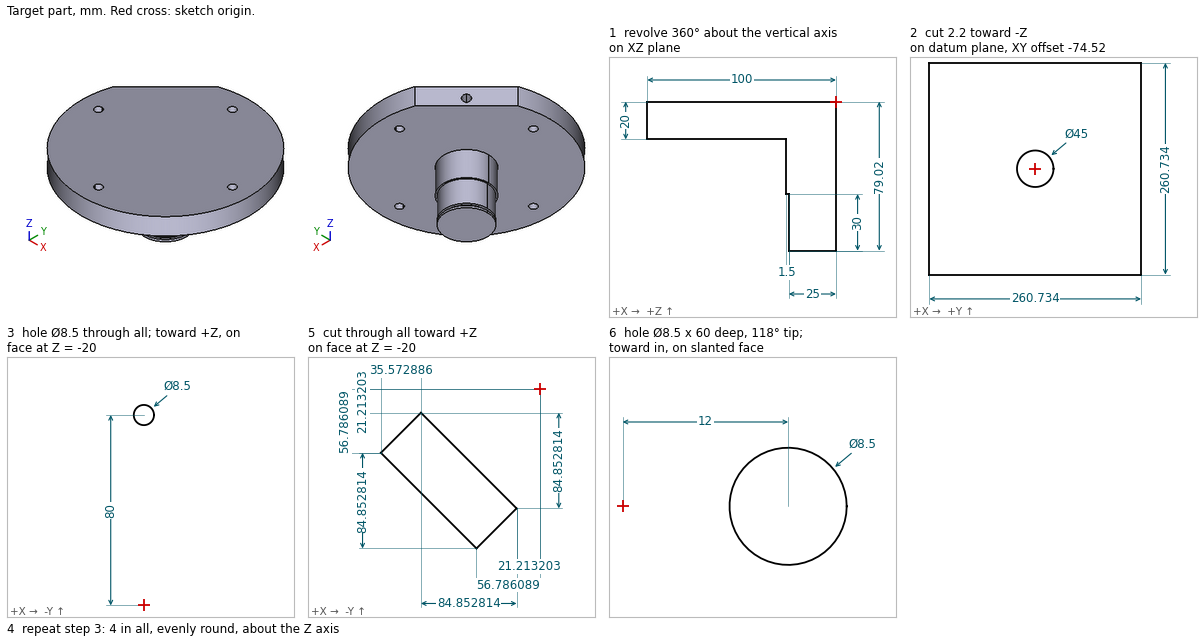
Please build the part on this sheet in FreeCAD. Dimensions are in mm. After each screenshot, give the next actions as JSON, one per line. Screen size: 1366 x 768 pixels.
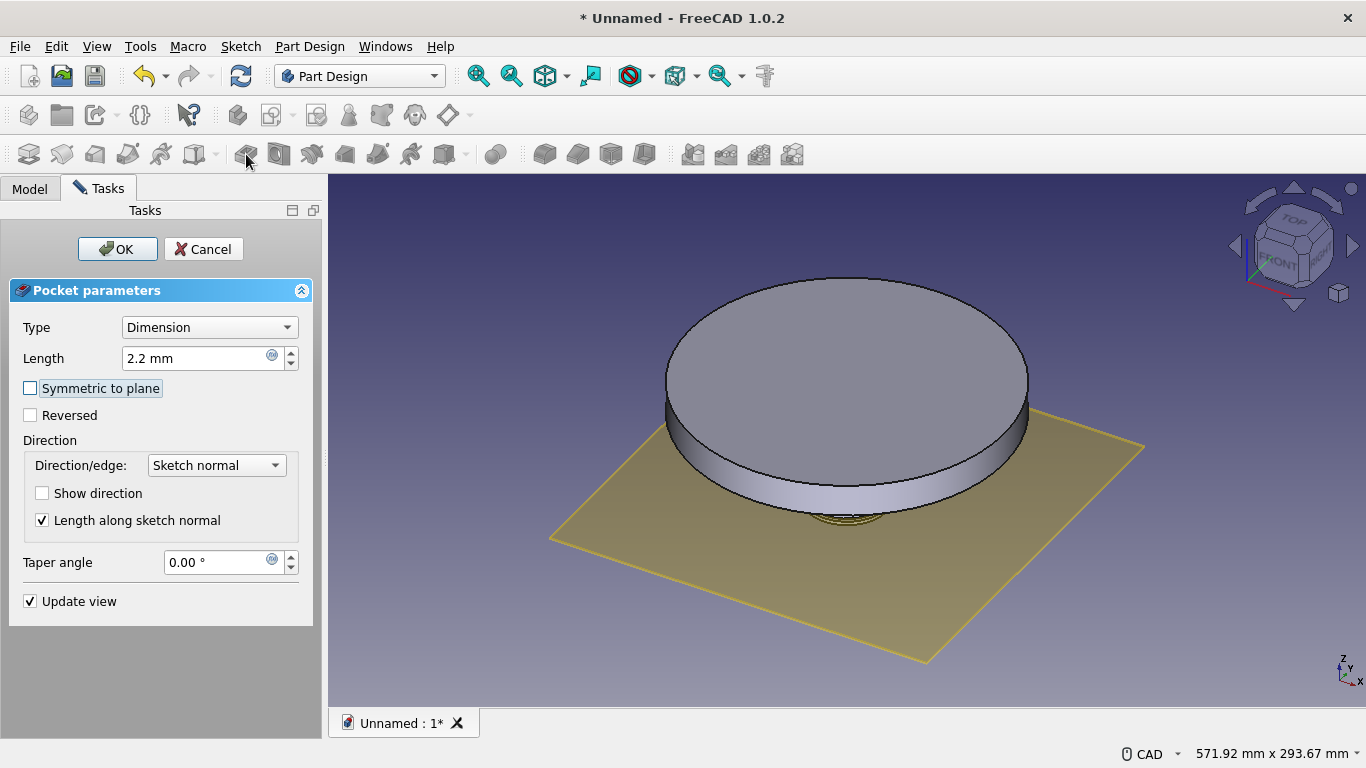
{"action": "left_click", "coordinate": [118, 249]}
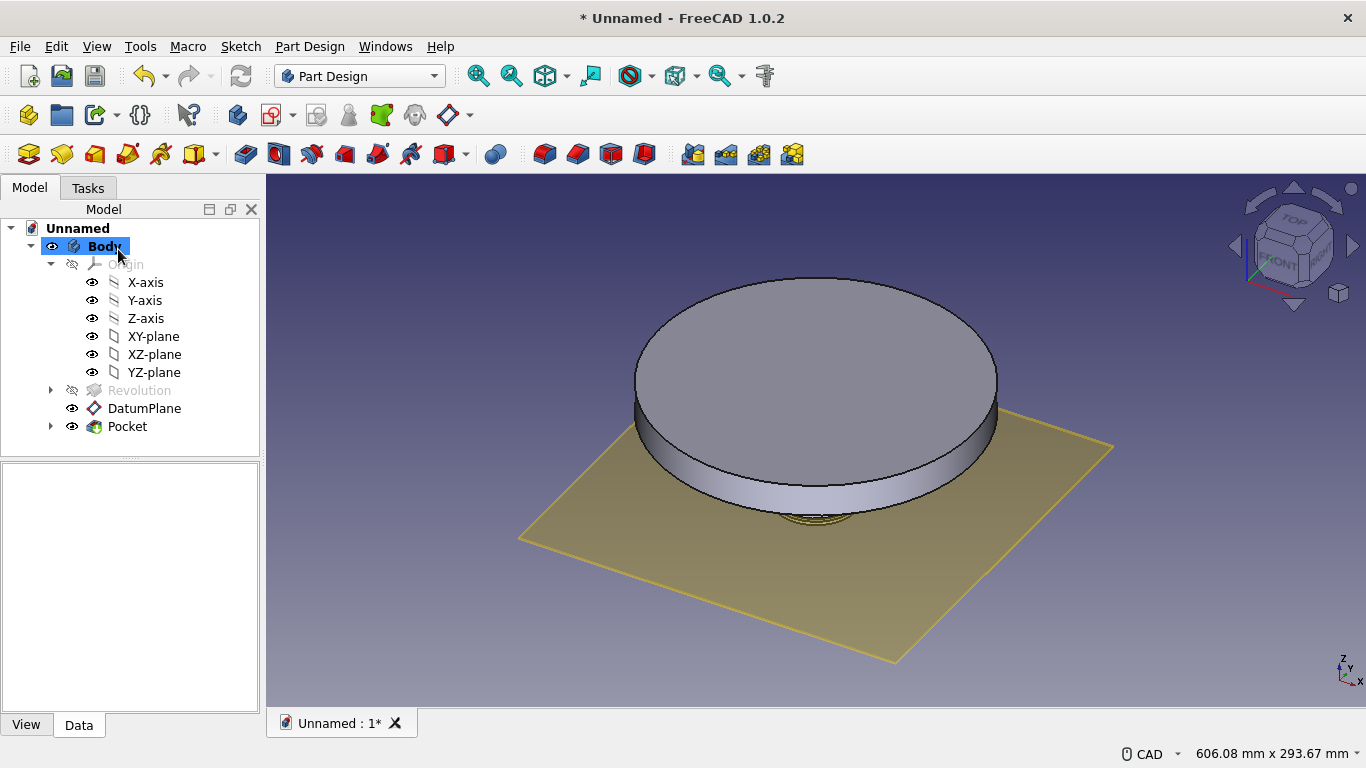
{"action": "left_click", "coordinate": [117, 408]}
{"action": "key", "text": "space"}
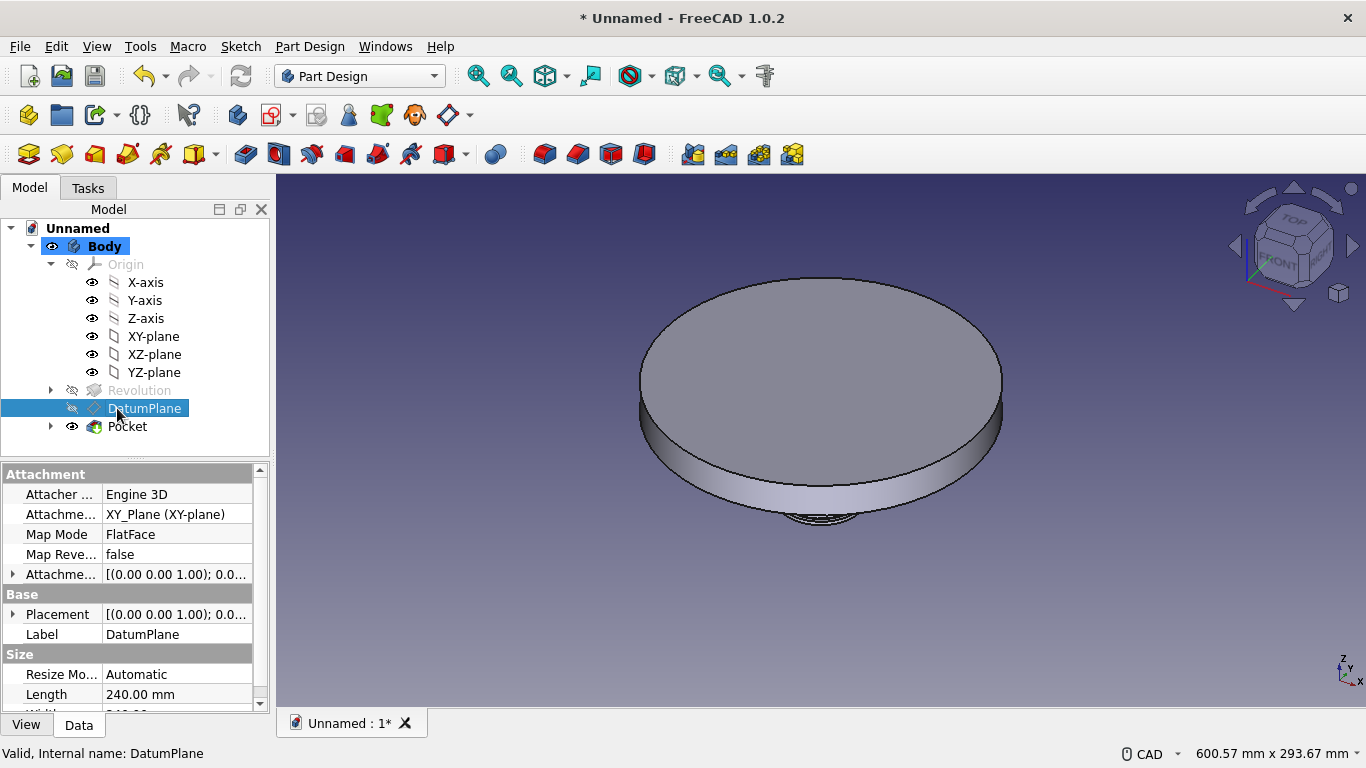
{"action": "key", "text": "5"}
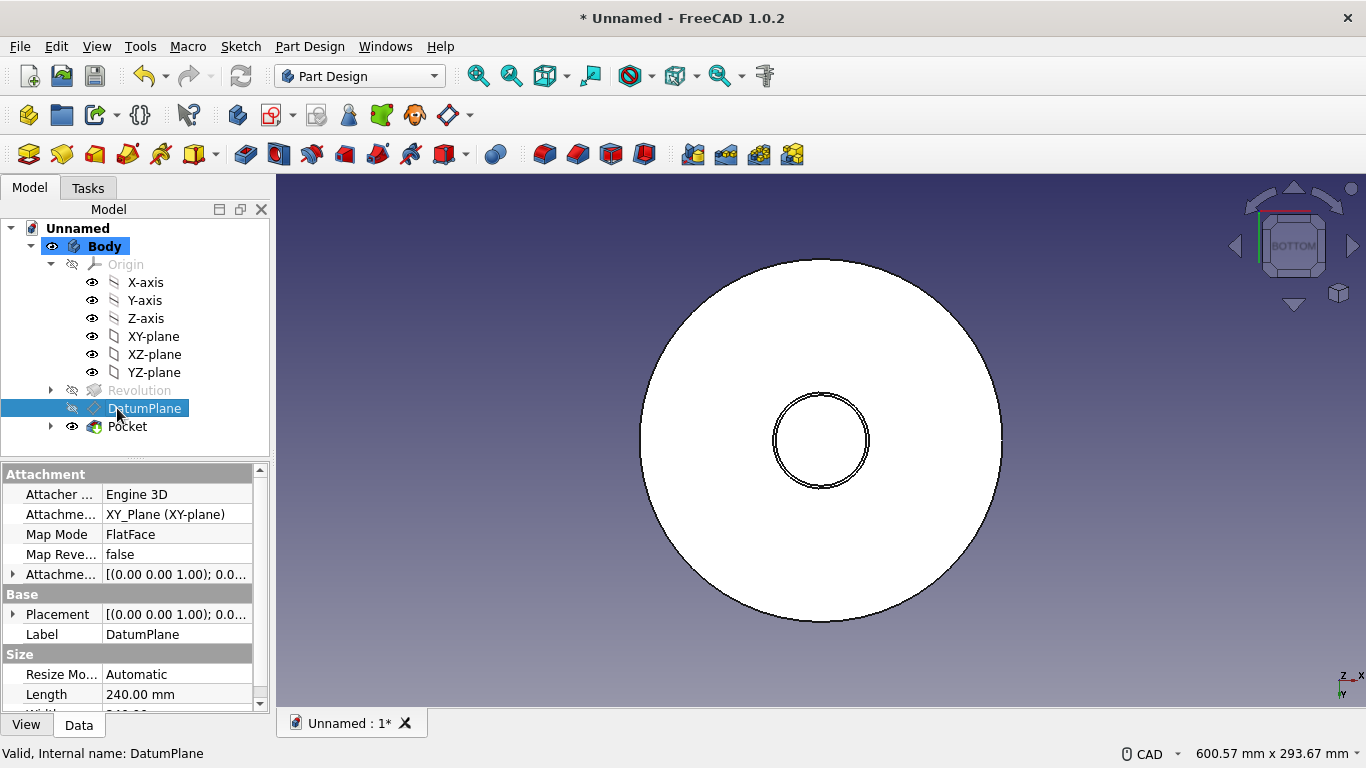
{"action": "left_click", "coordinate": [925, 491]}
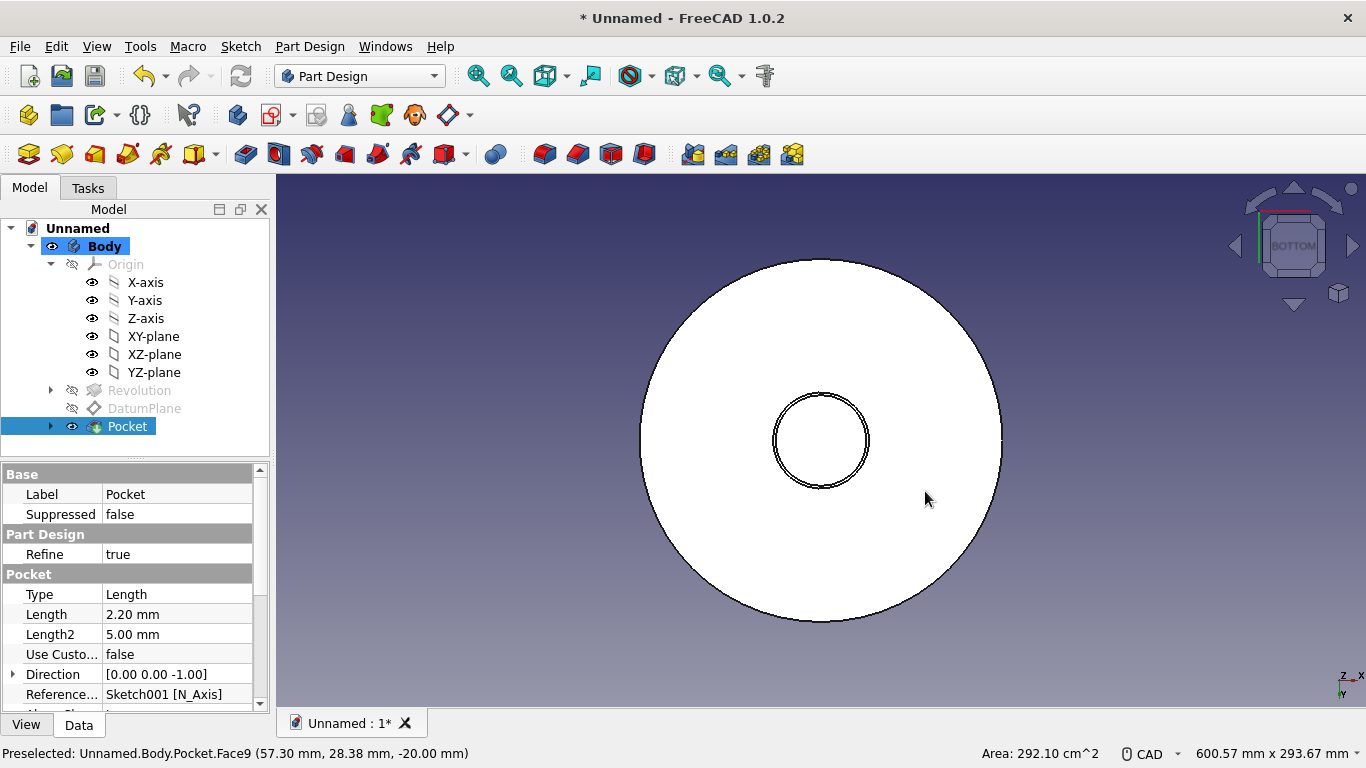
{"action": "left_click", "coordinate": [270, 116]}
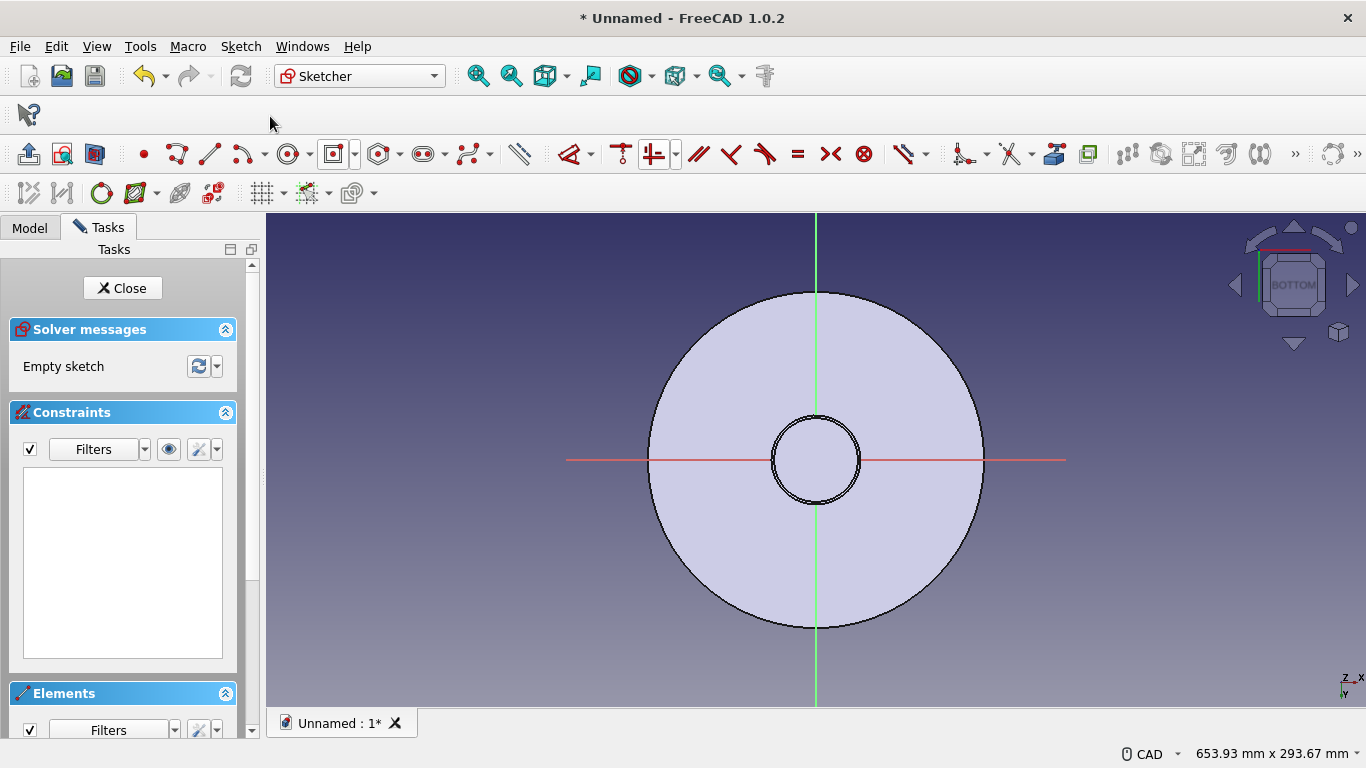
{"action": "left_click", "coordinate": [95, 154]}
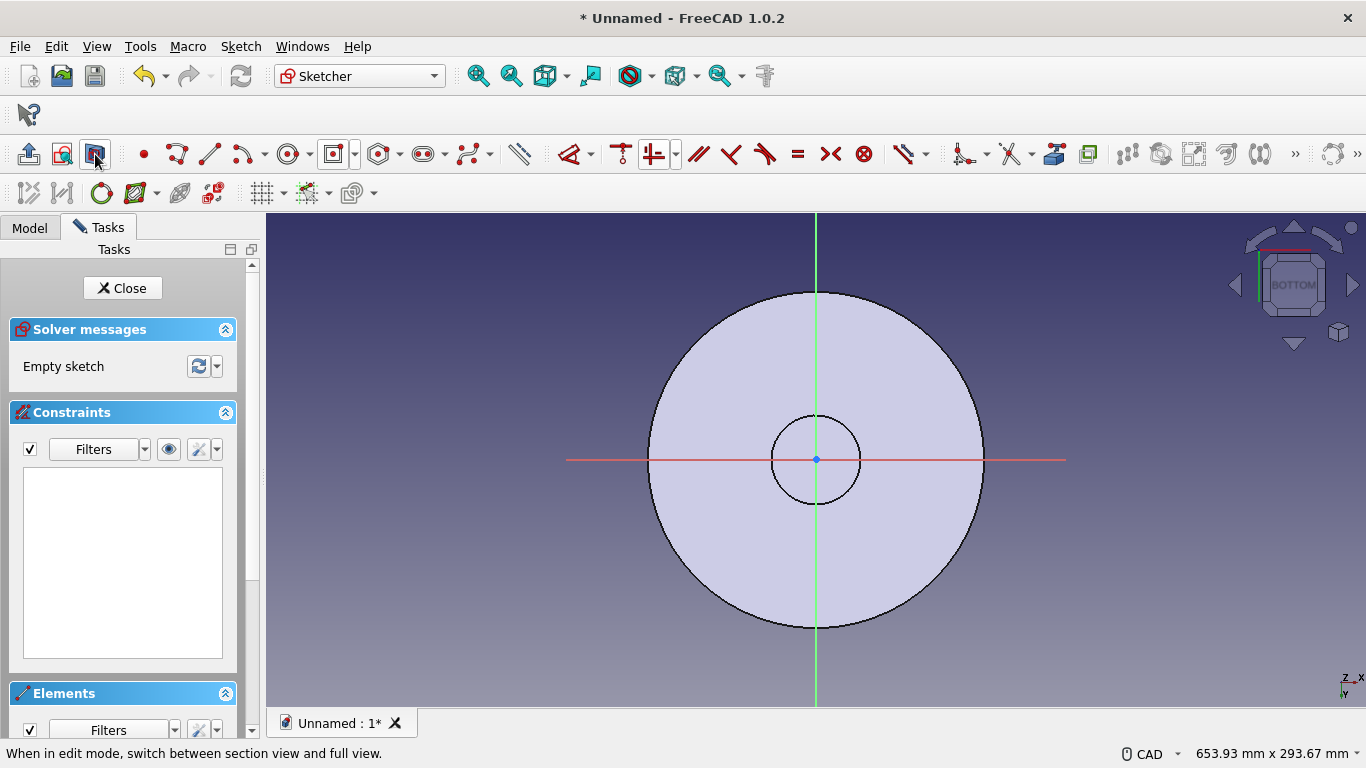
{"action": "scroll", "coordinate": [820, 318], "scroll_direction": "up", "scroll_amount": 15}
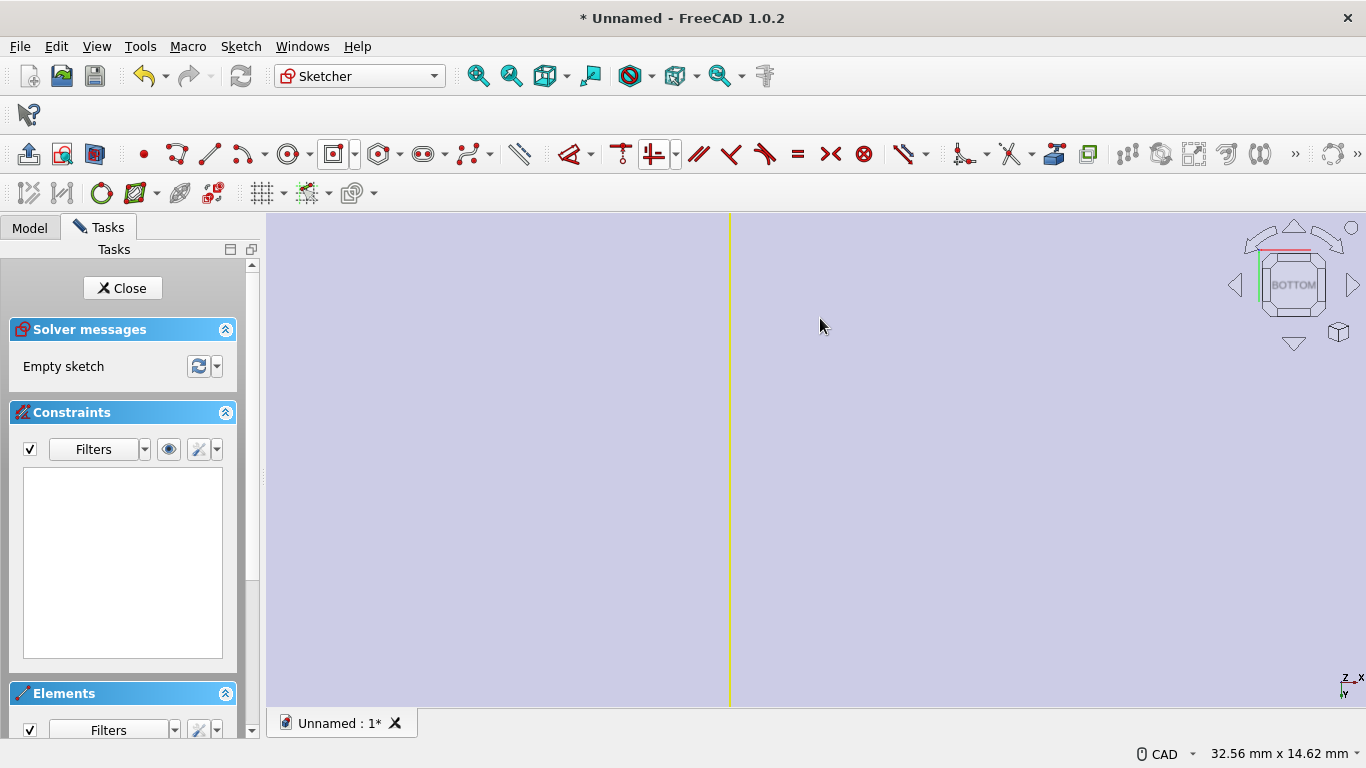
{"action": "left_click", "coordinate": [288, 154]}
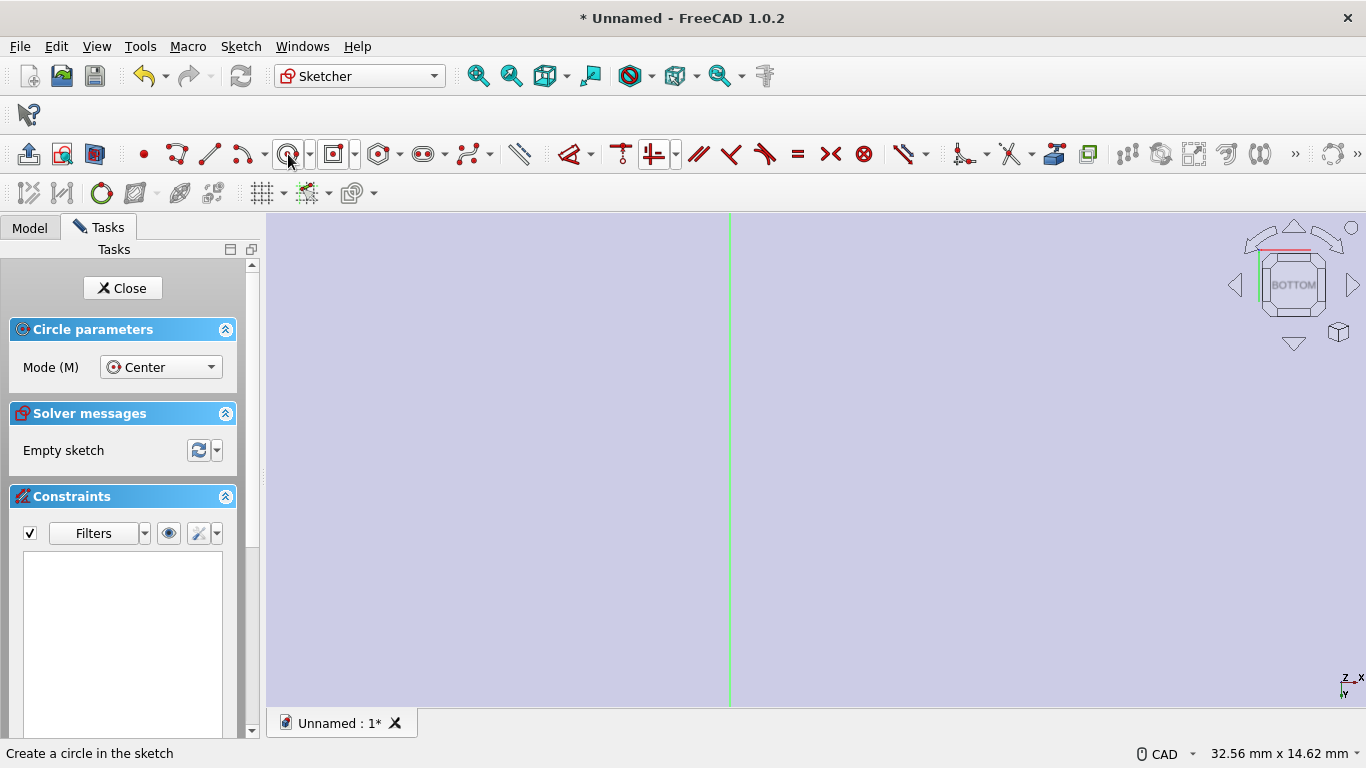
{"action": "left_click", "coordinate": [730, 463]}
{"action": "mouse_move", "coordinate": [832, 362]}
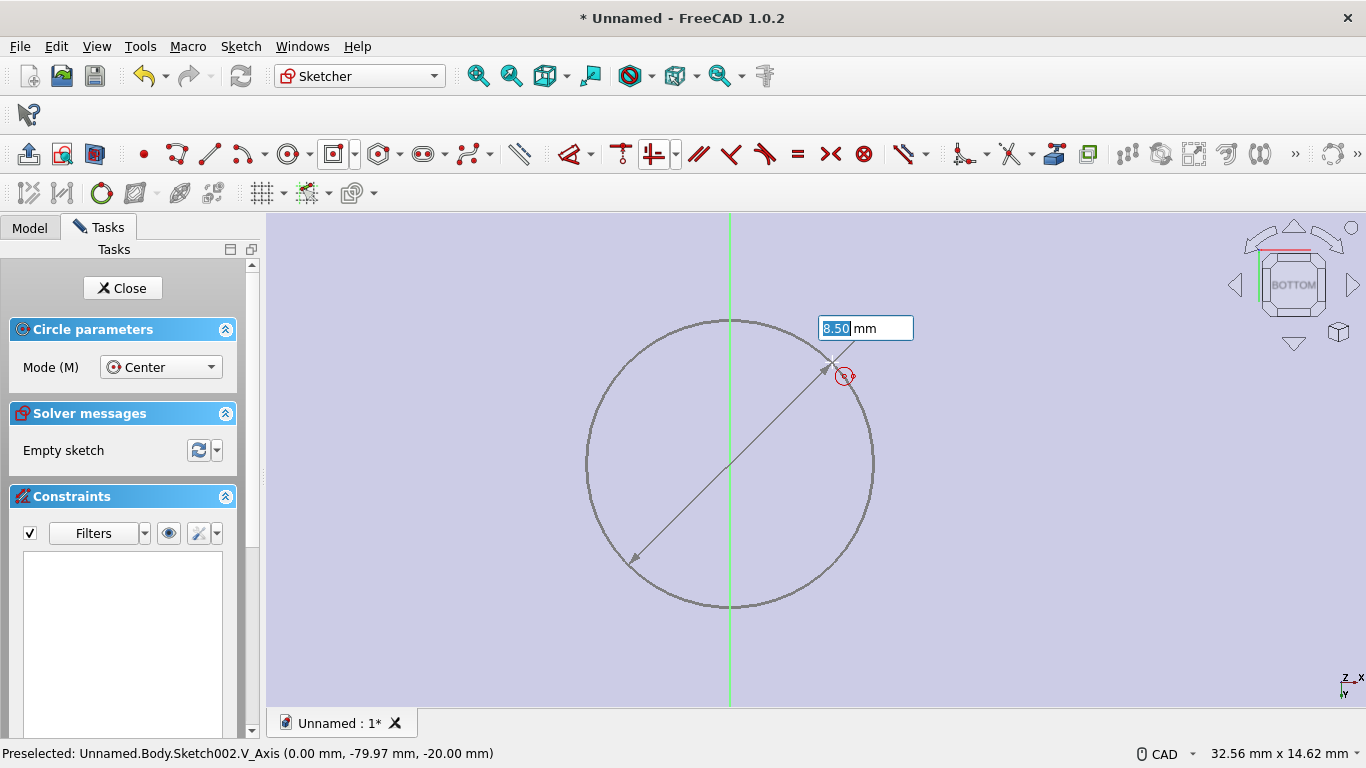
{"action": "type", "text": "8.5"}
{"action": "key", "text": "Return"}
{"action": "key", "text": "Escape"}